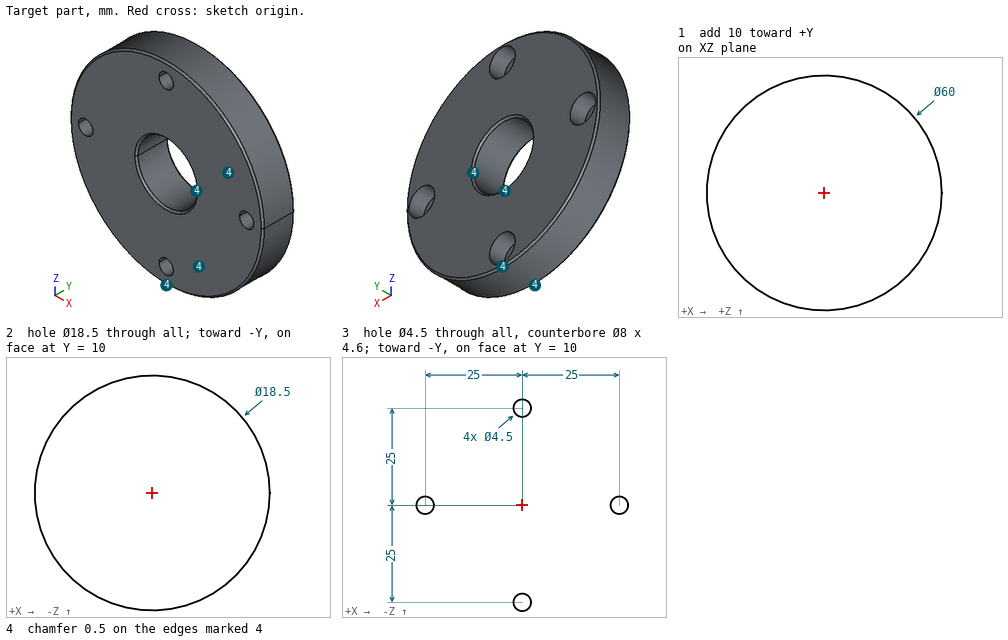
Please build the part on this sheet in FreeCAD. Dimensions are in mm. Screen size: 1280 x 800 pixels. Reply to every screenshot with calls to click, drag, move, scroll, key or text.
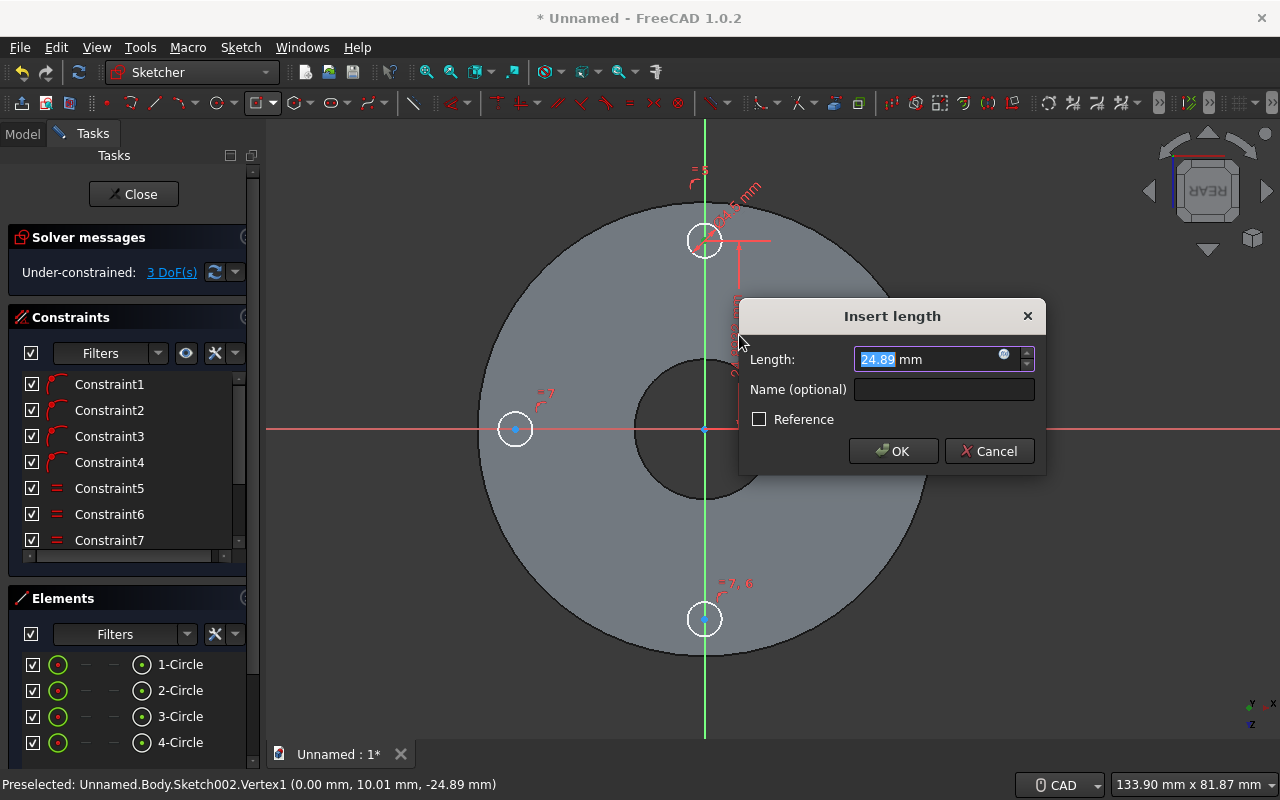
text(25)
key(Return)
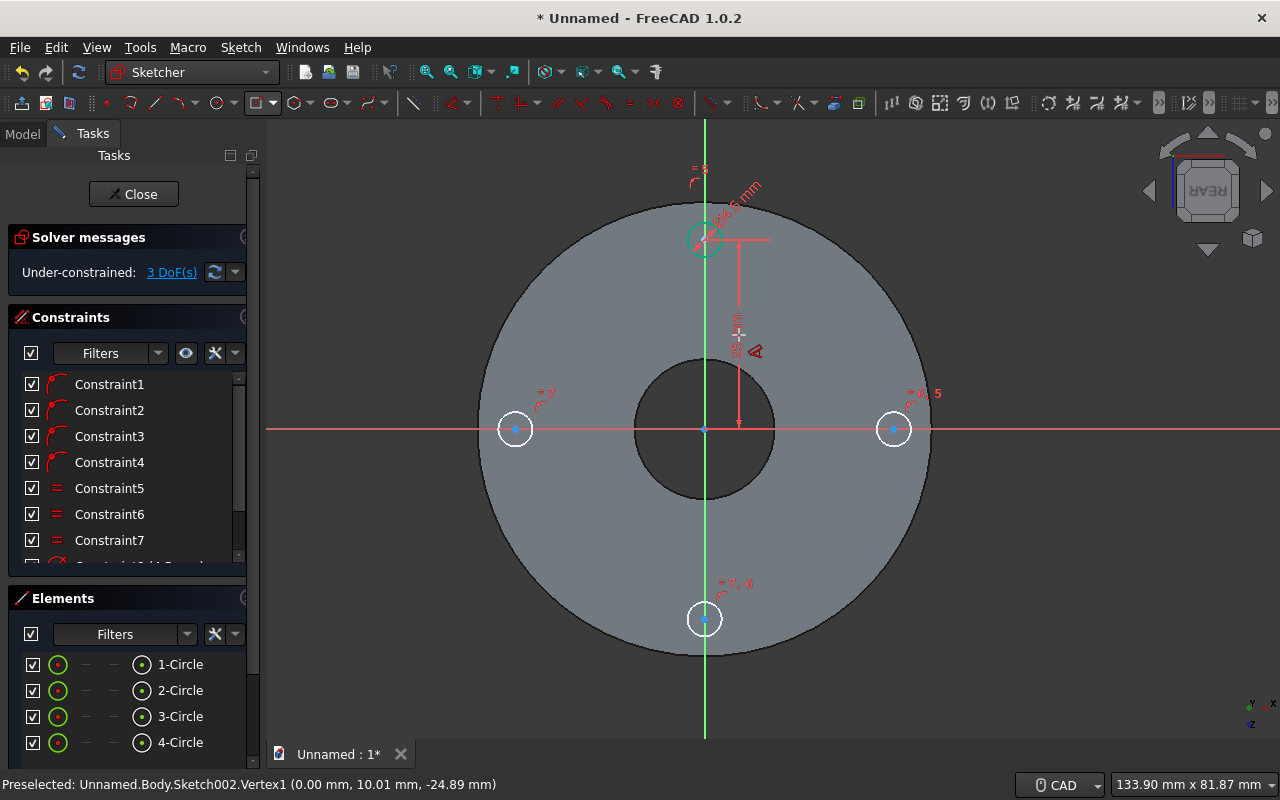
click(894, 429)
click(799, 463)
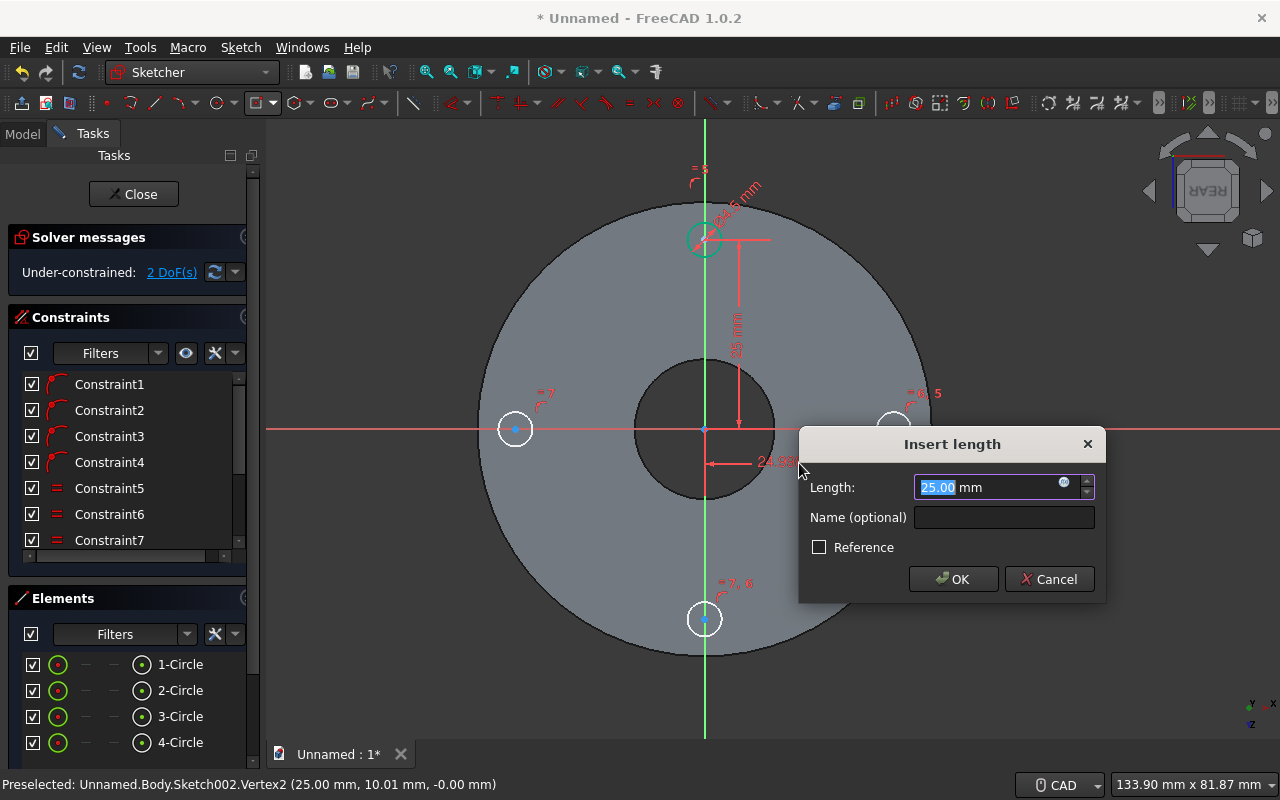
text(25)
key(Return)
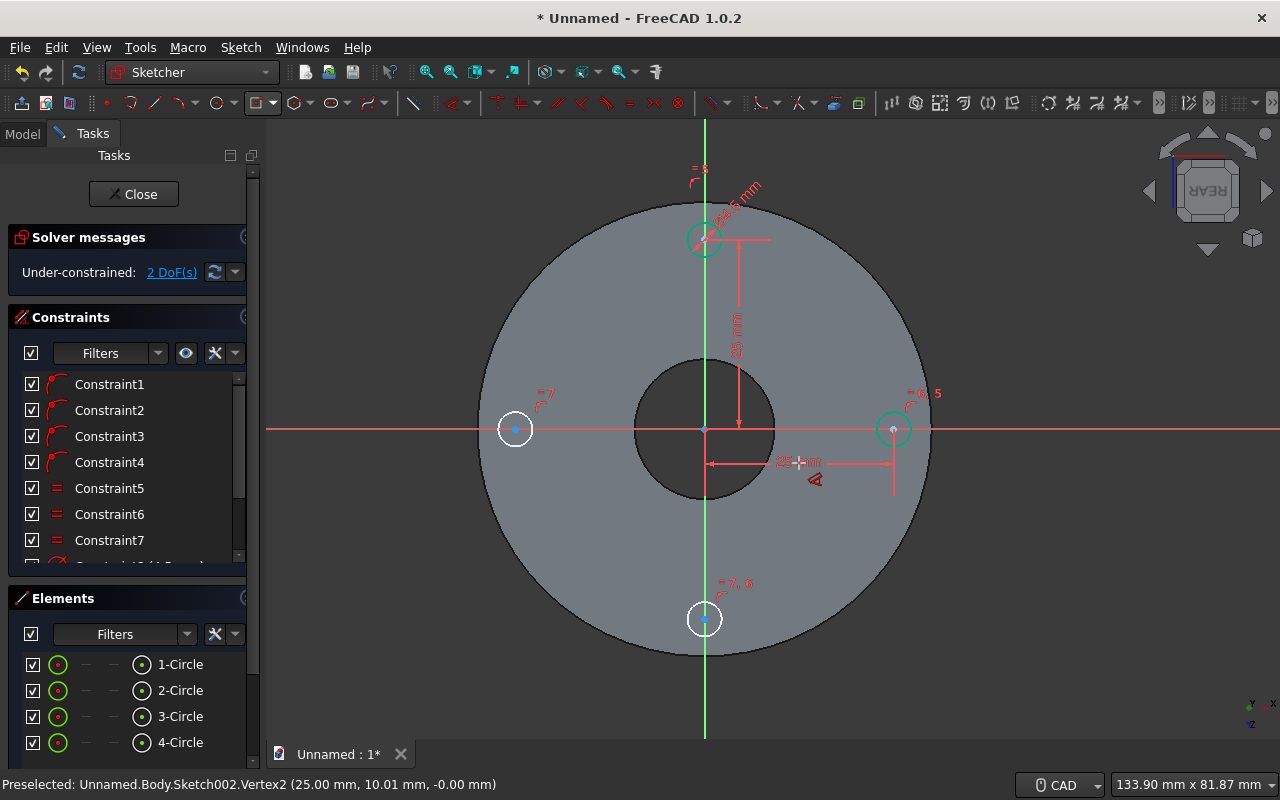
click(705, 619)
click(739, 524)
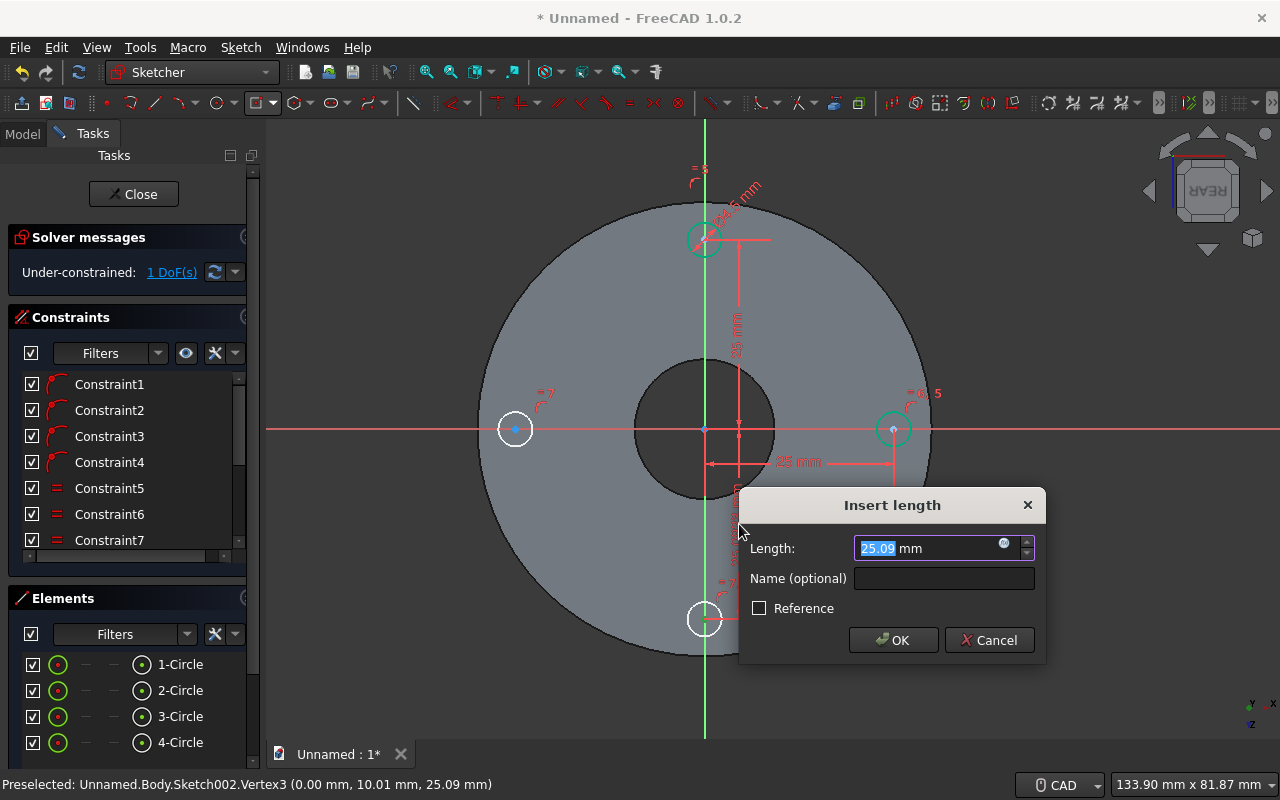
text(25)
key(Return)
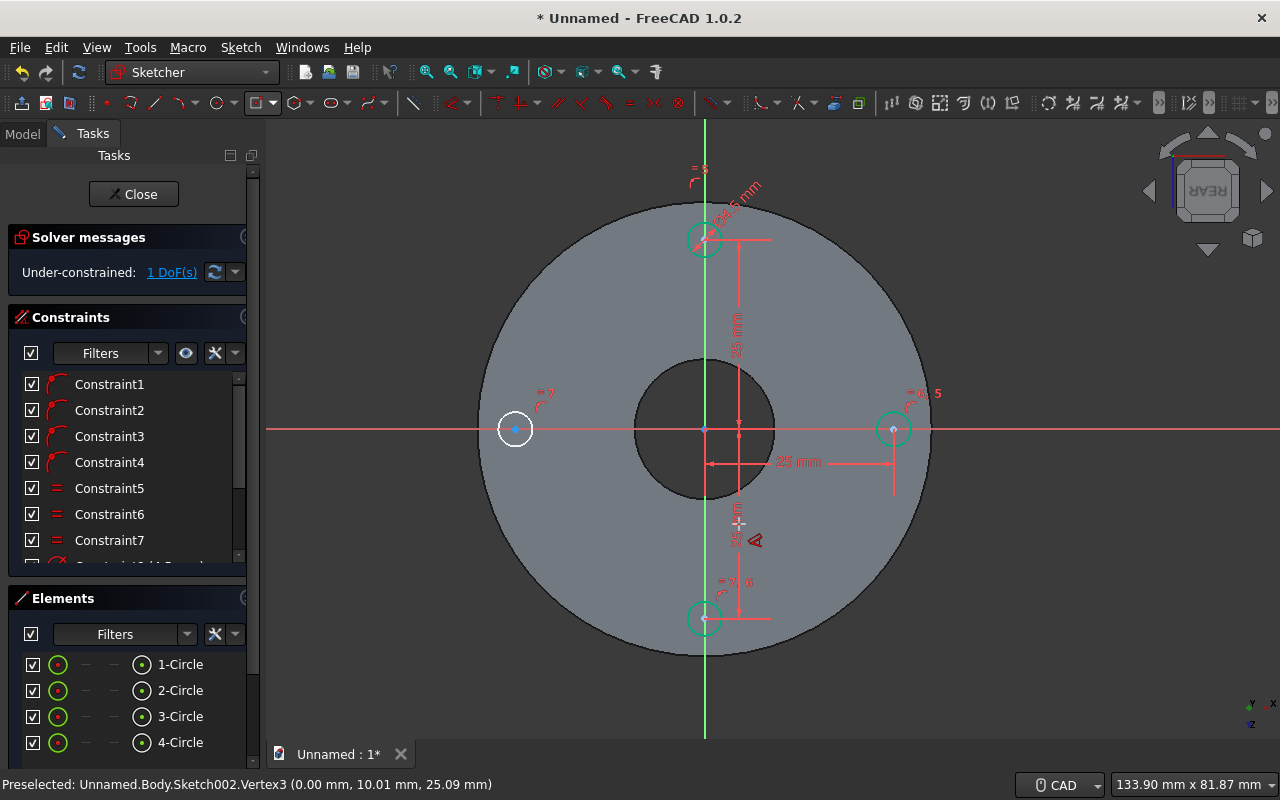
click(515, 429)
click(610, 463)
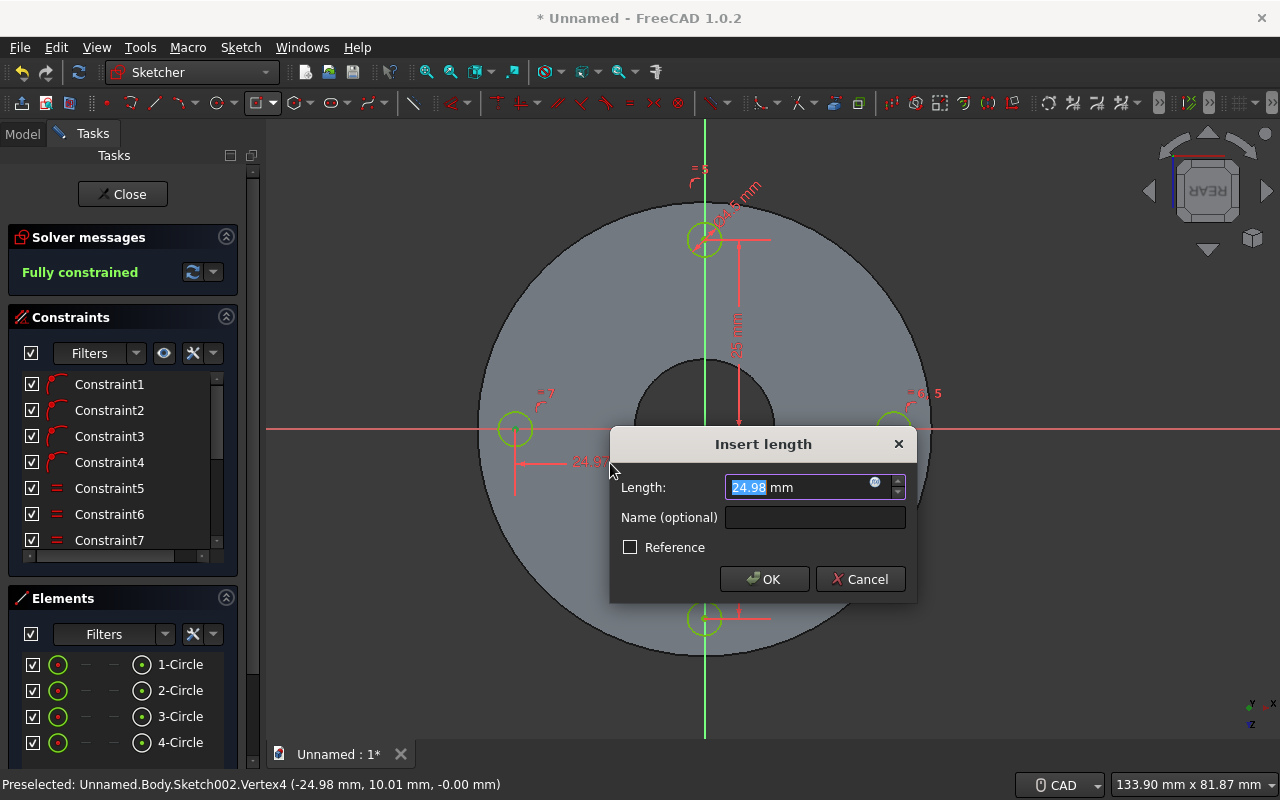
text(25)
key(Return)
key(Escape)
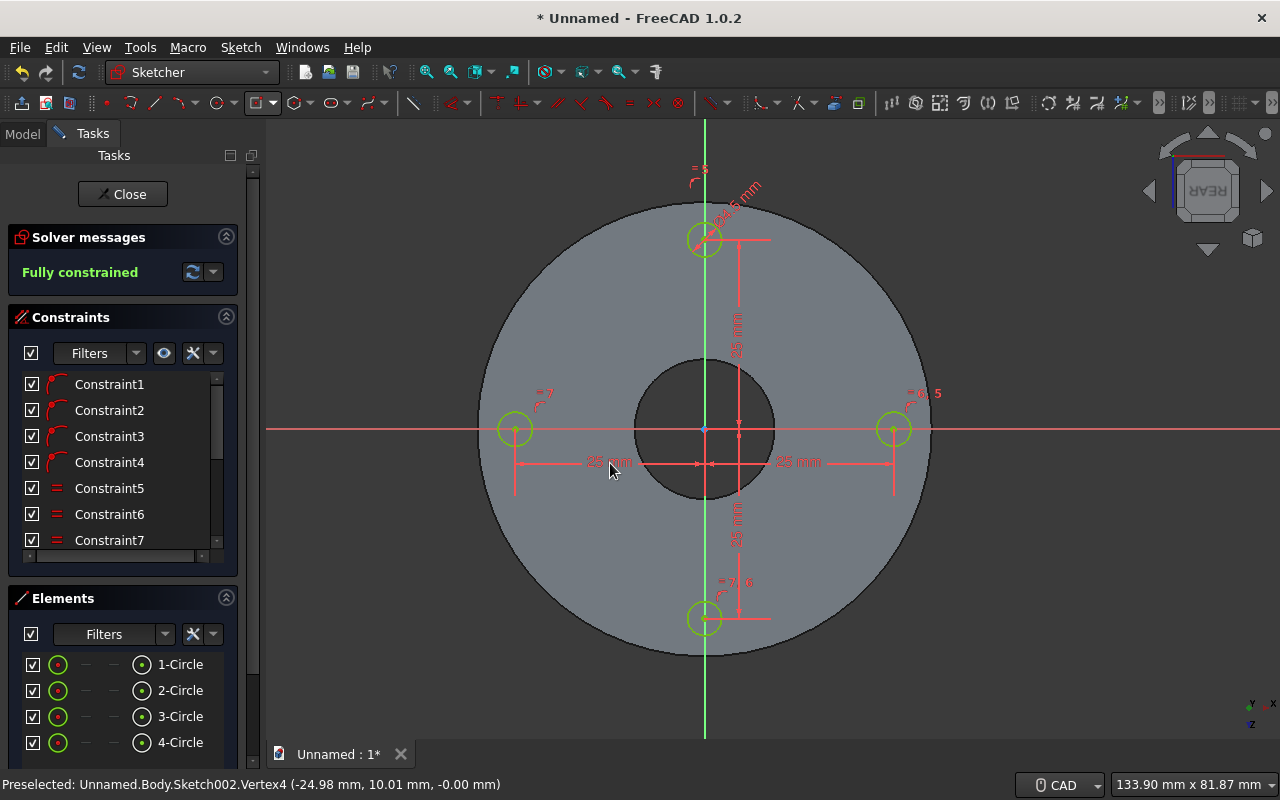
click(123, 194)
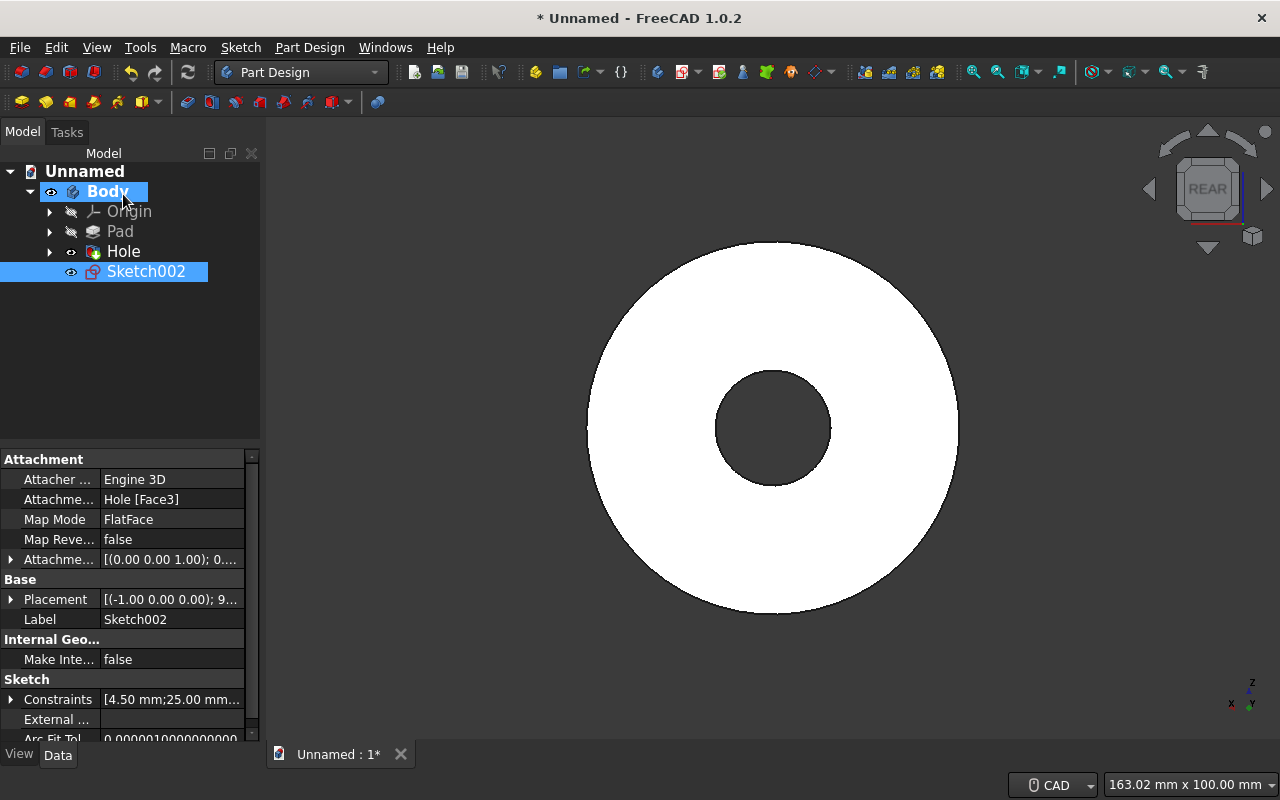
click(212, 102)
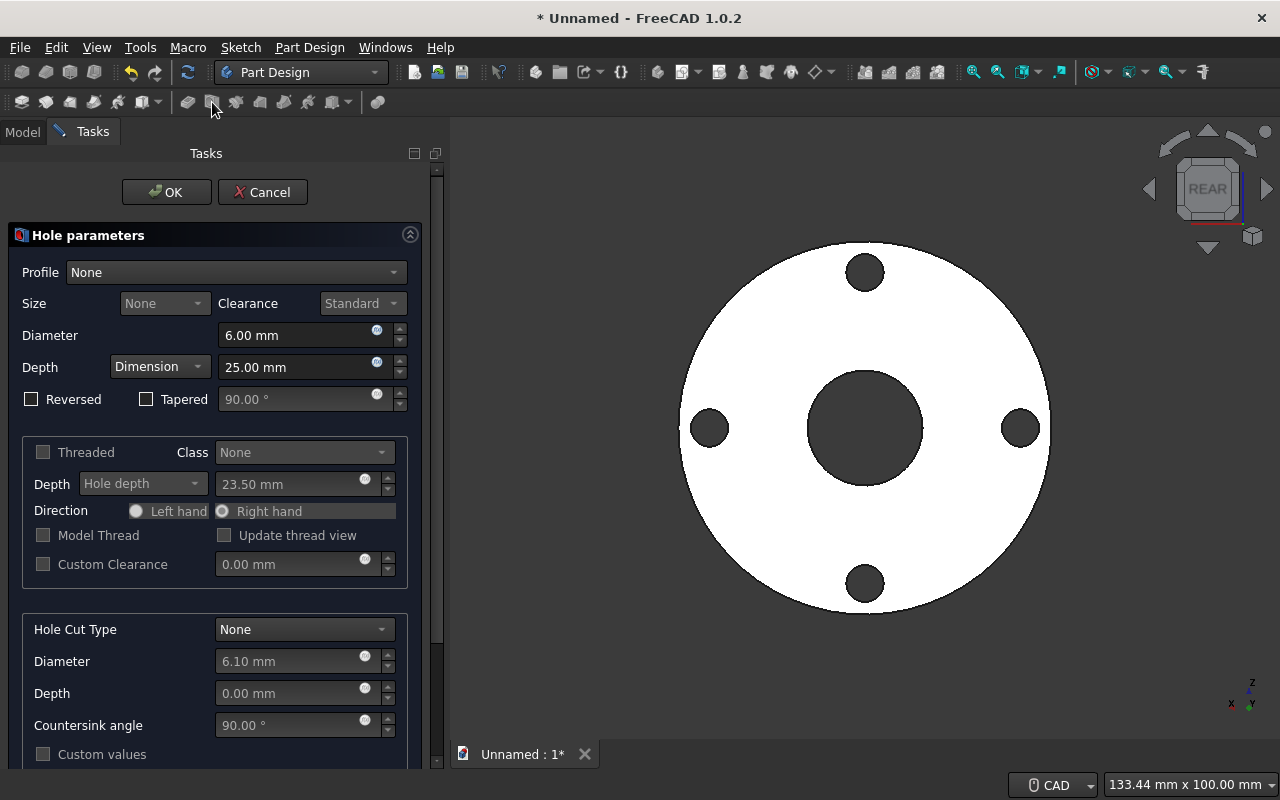
triple_click(305, 335)